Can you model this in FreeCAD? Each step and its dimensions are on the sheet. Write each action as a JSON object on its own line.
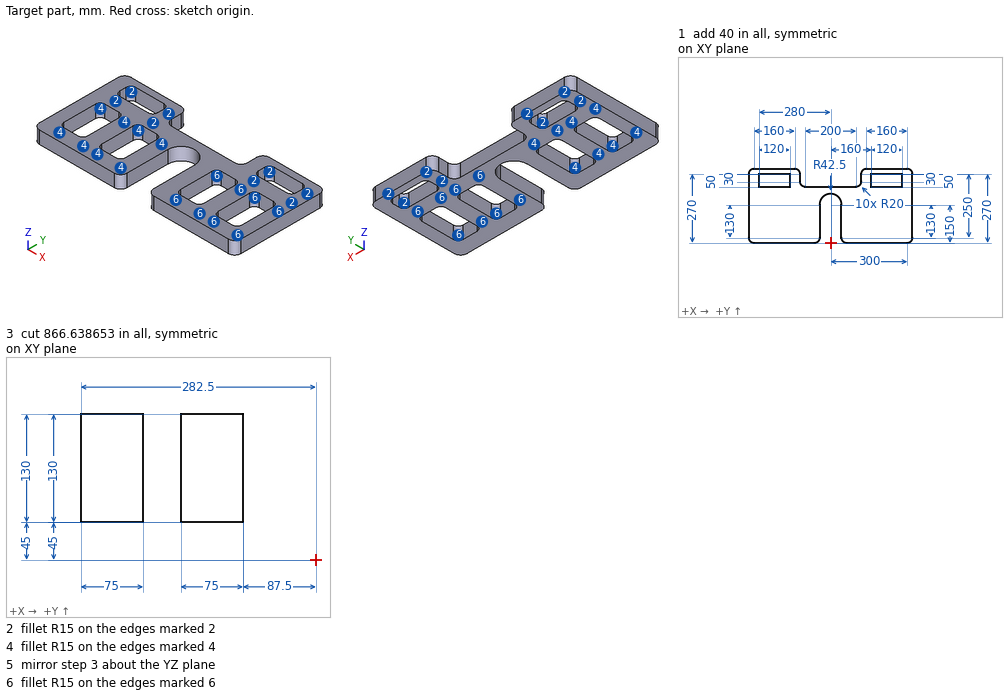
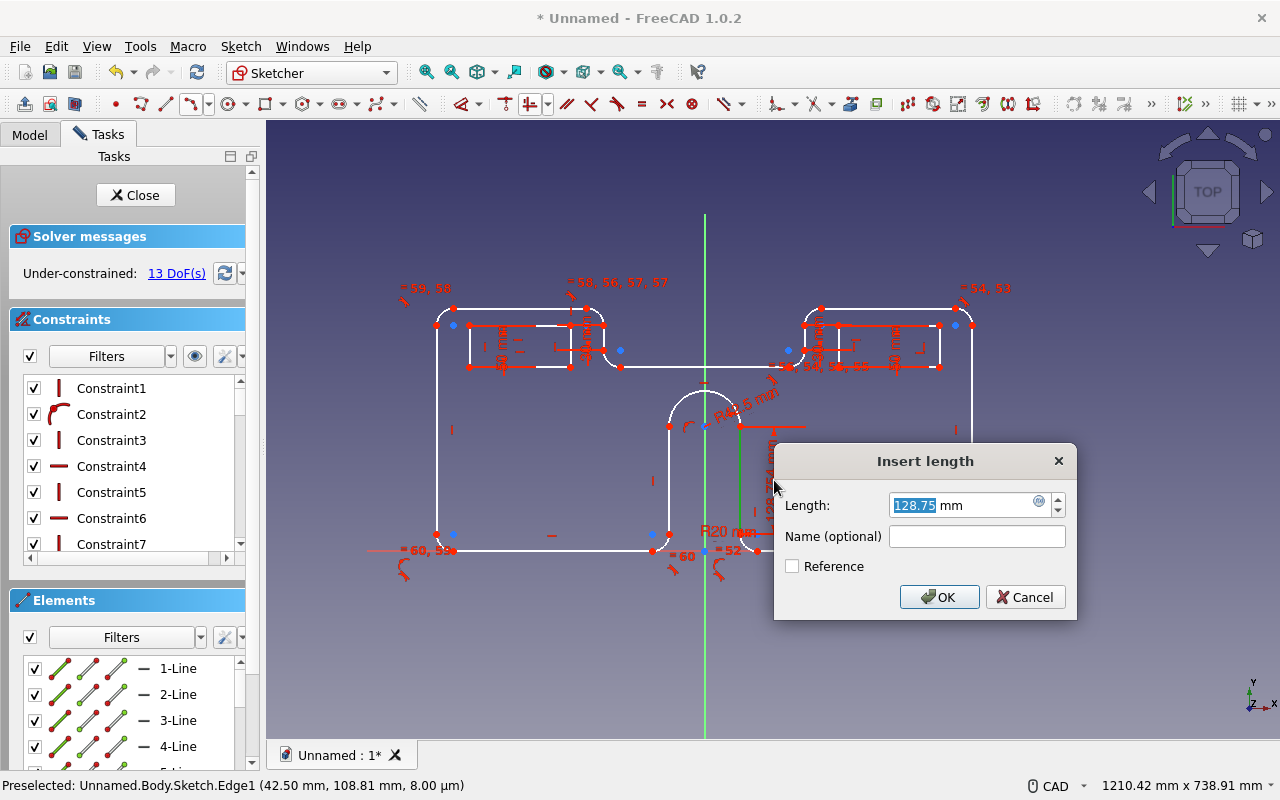
{"action": "type", "text": "130"}
{"action": "key", "text": "Return"}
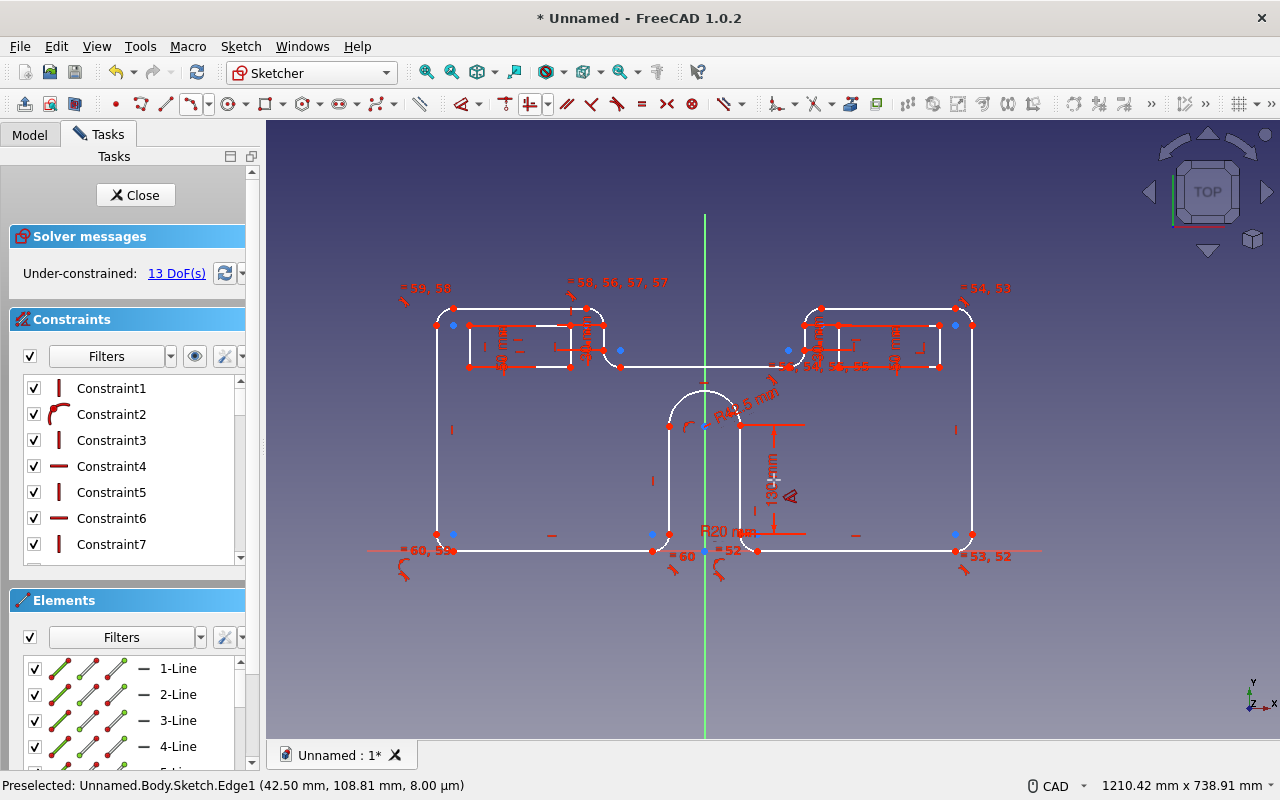
{"action": "left_click", "coordinate": [972, 472]}
{"action": "left_click", "coordinate": [1006, 430]}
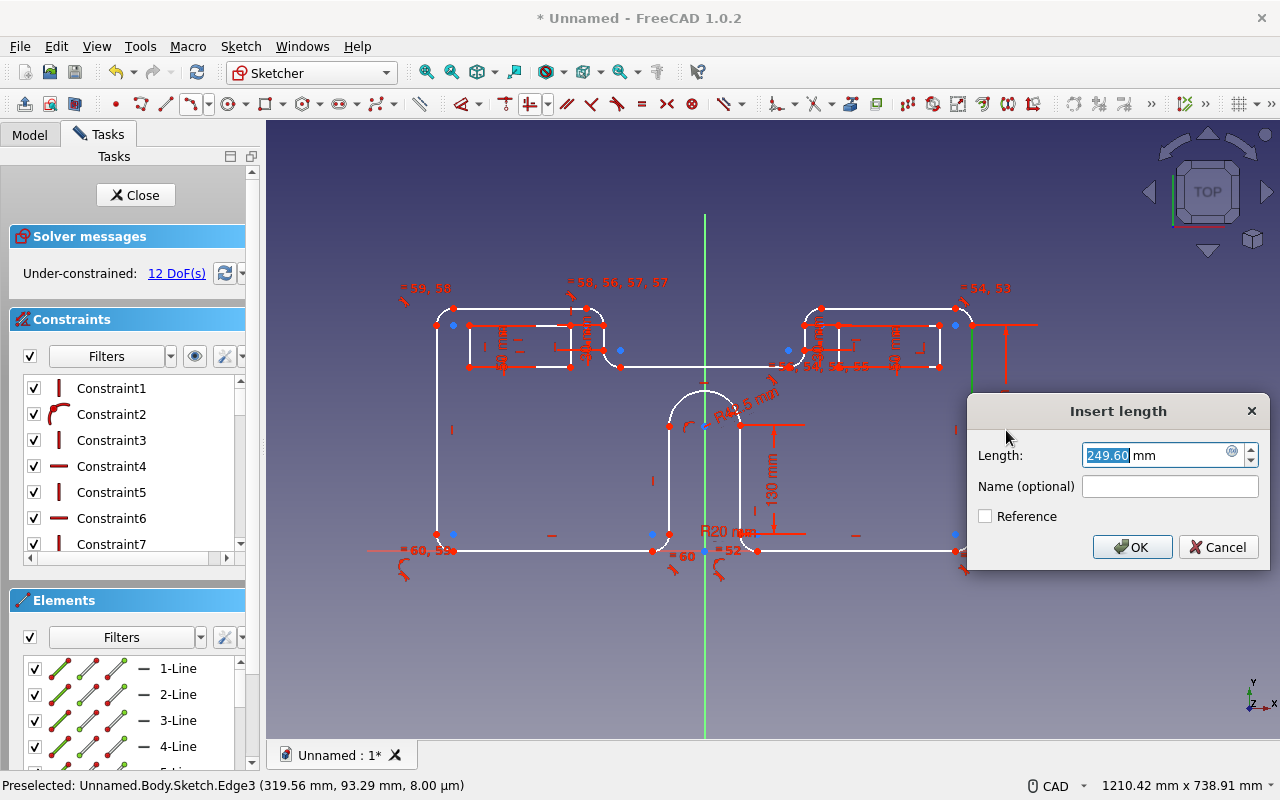
{"action": "type", "text": "250"}
{"action": "key", "text": "Return"}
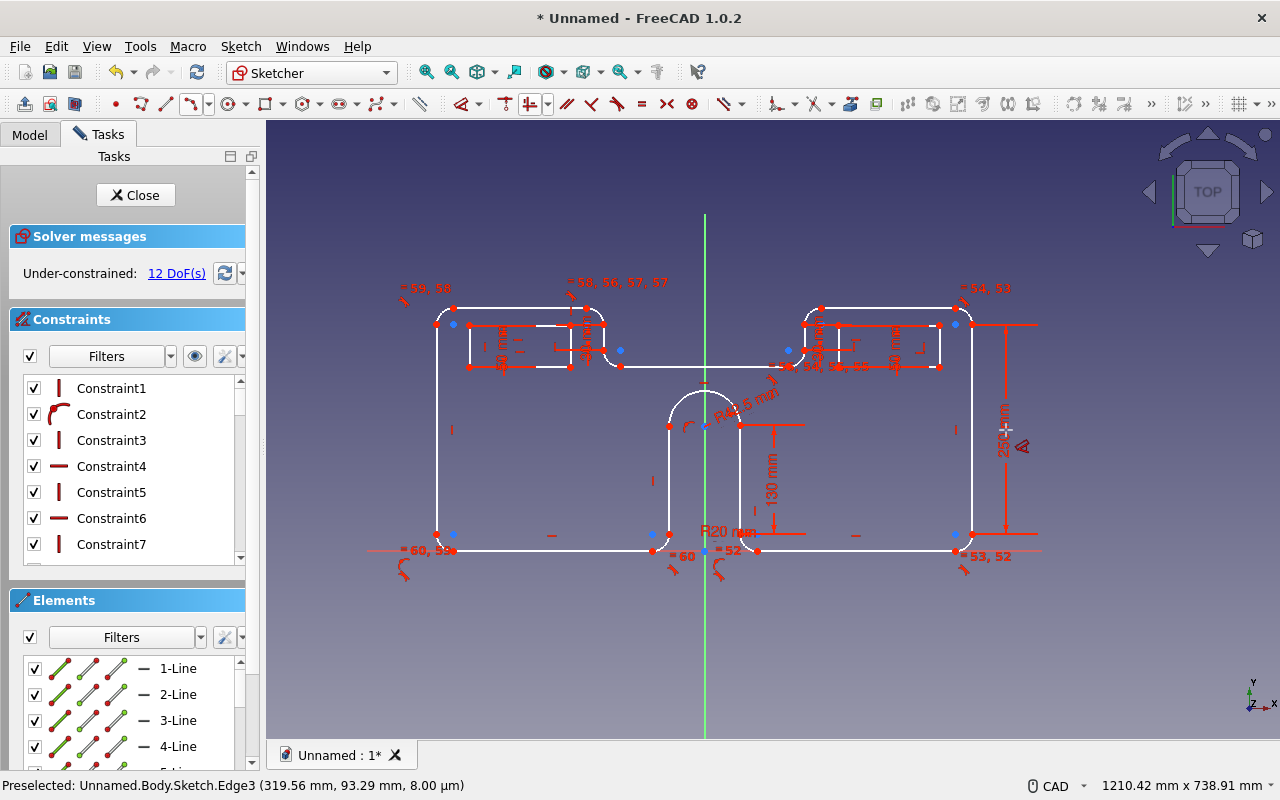
{"action": "left_click", "coordinate": [915, 308]}
{"action": "left_click", "coordinate": [889, 274]}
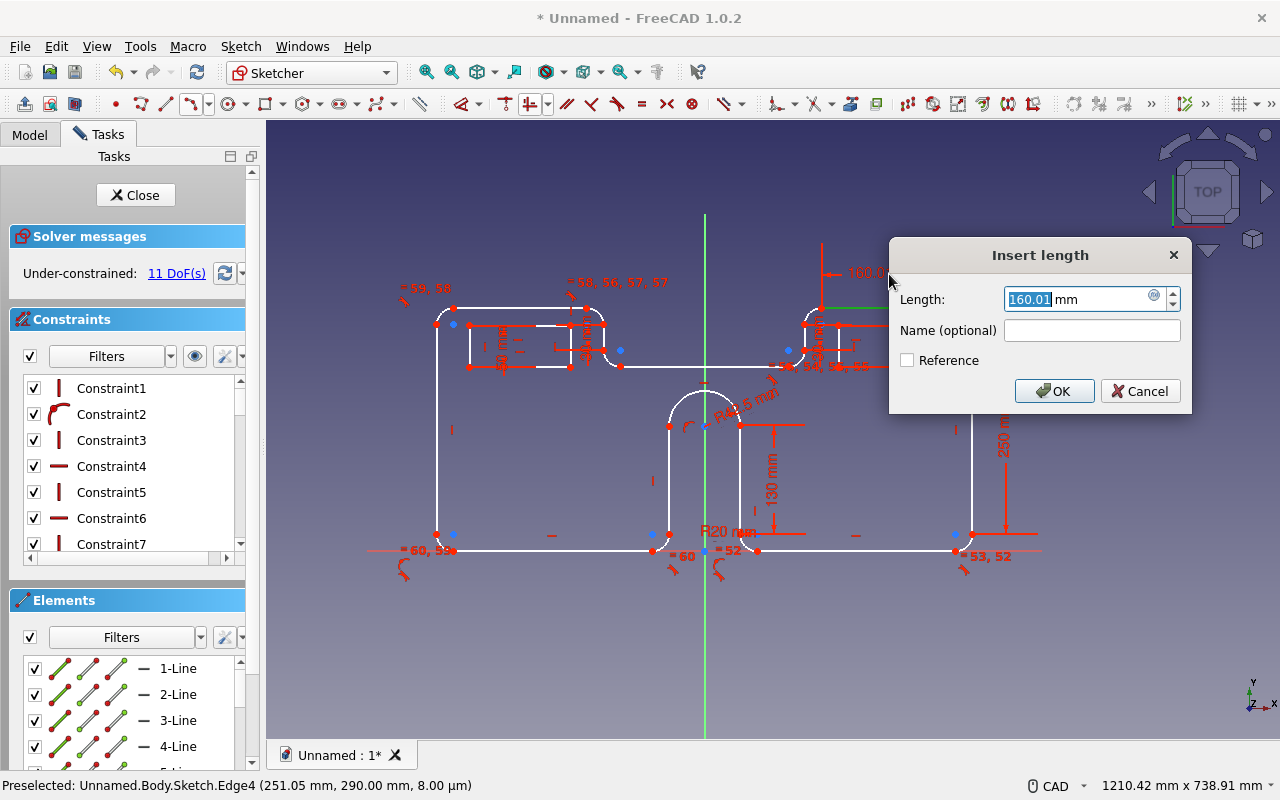
{"action": "type", "text": "160"}
{"action": "key", "text": "Return"}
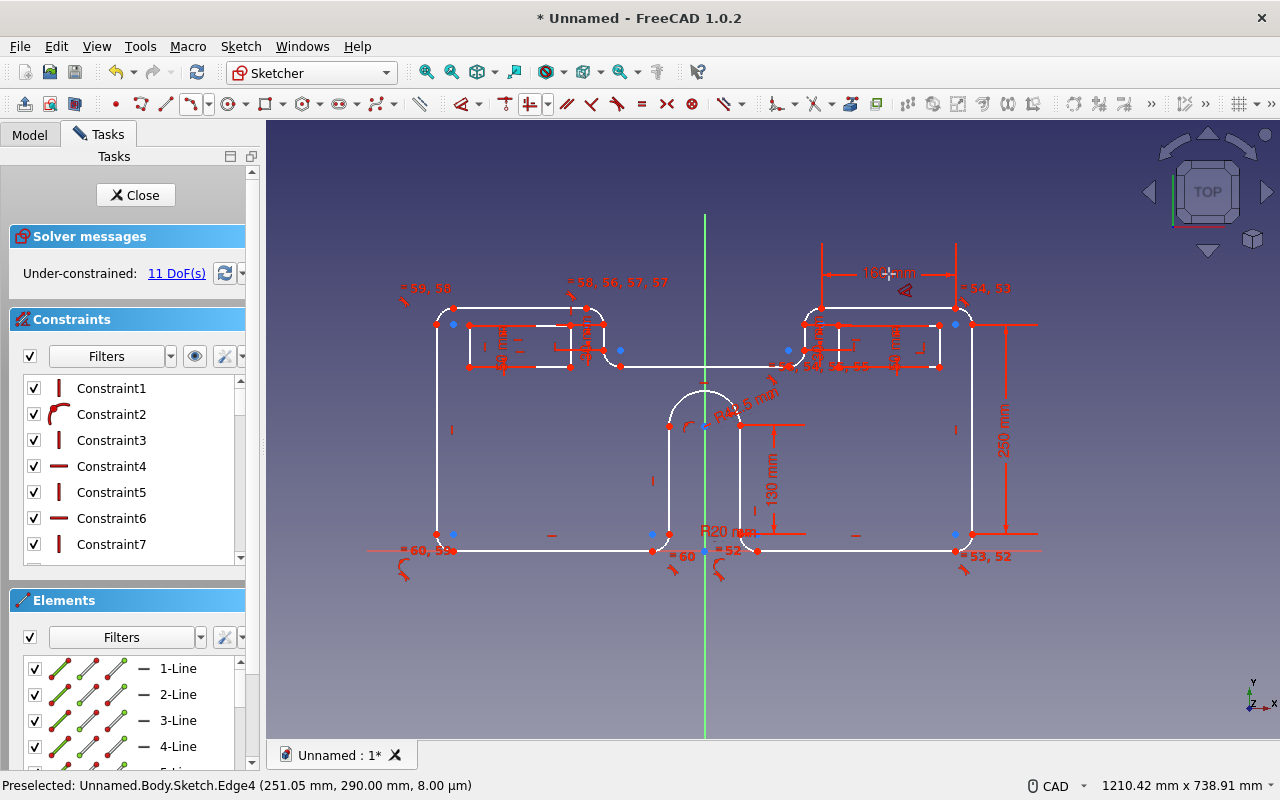
{"action": "left_click", "coordinate": [738, 367]}
{"action": "left_click", "coordinate": [666, 333]}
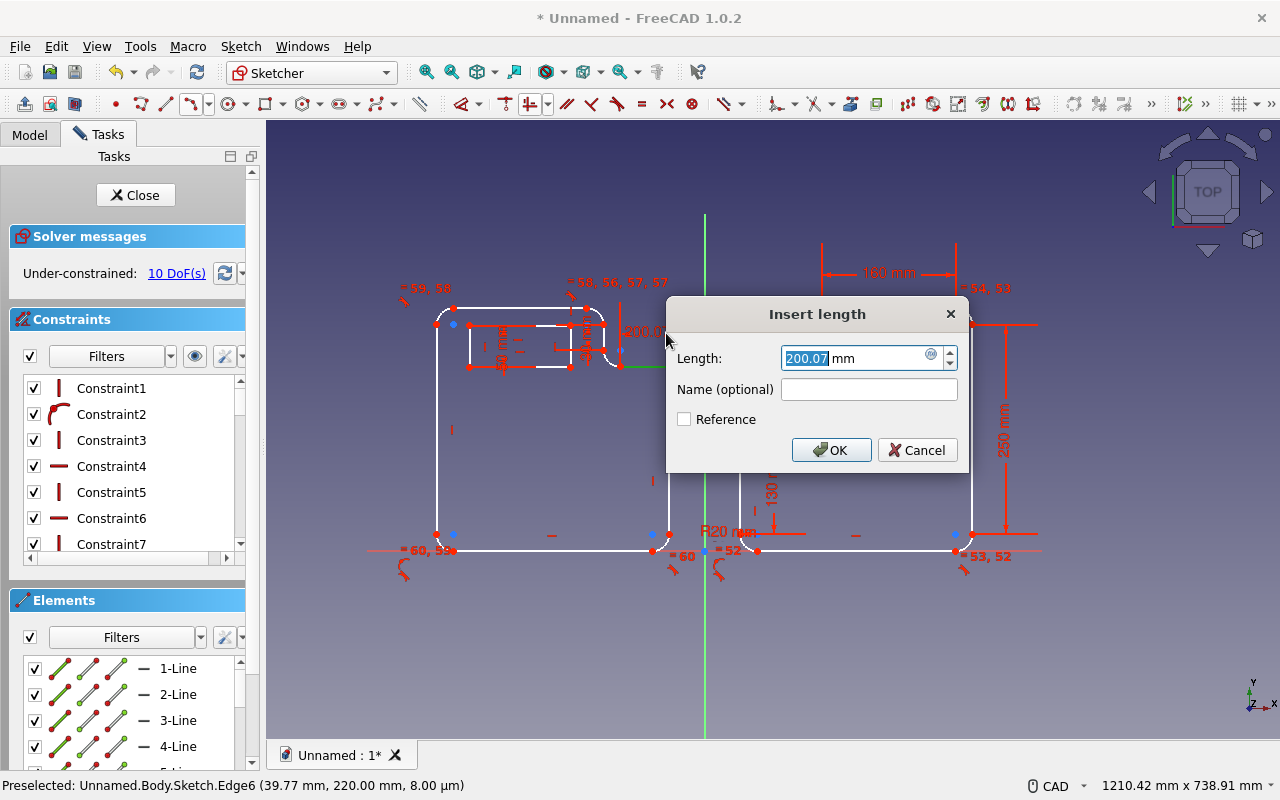
{"action": "type", "text": "200"}
{"action": "key", "text": "Return"}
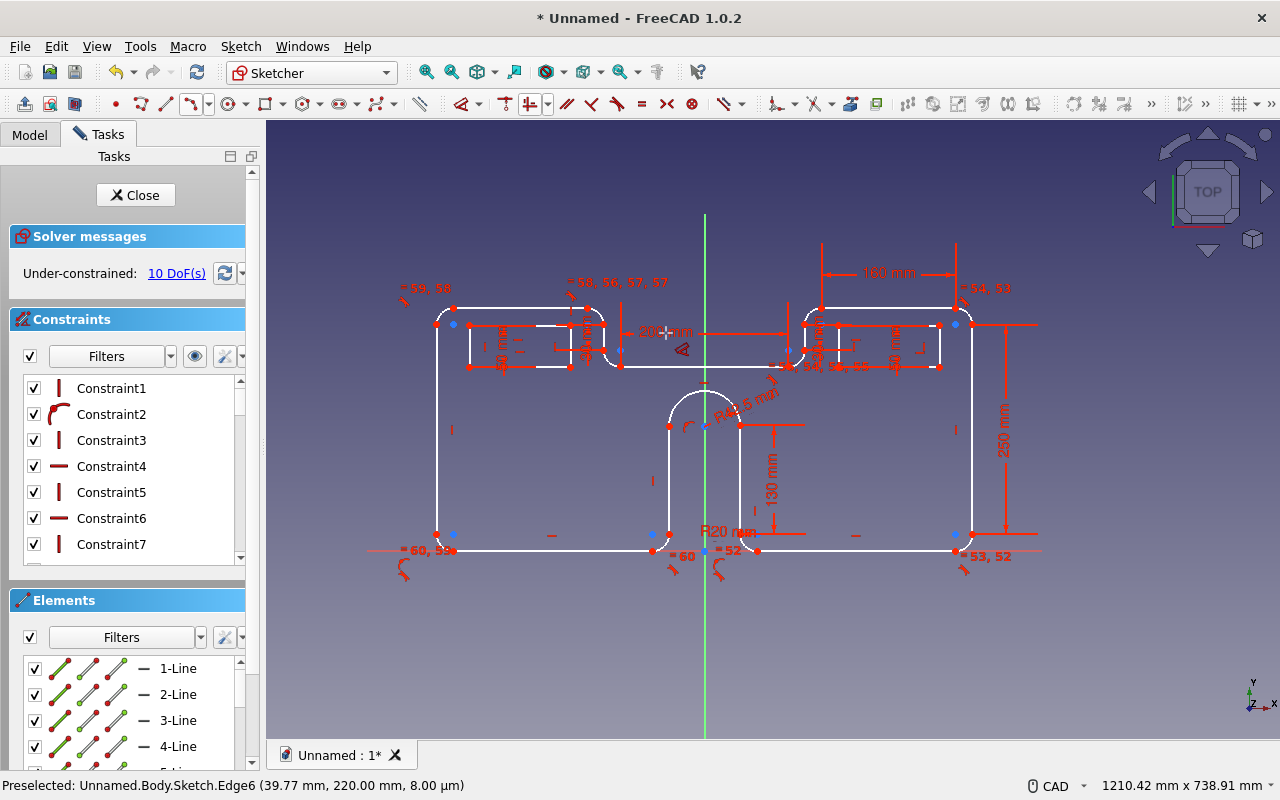
{"action": "left_click", "coordinate": [547, 308]}
{"action": "left_click", "coordinate": [520, 274]}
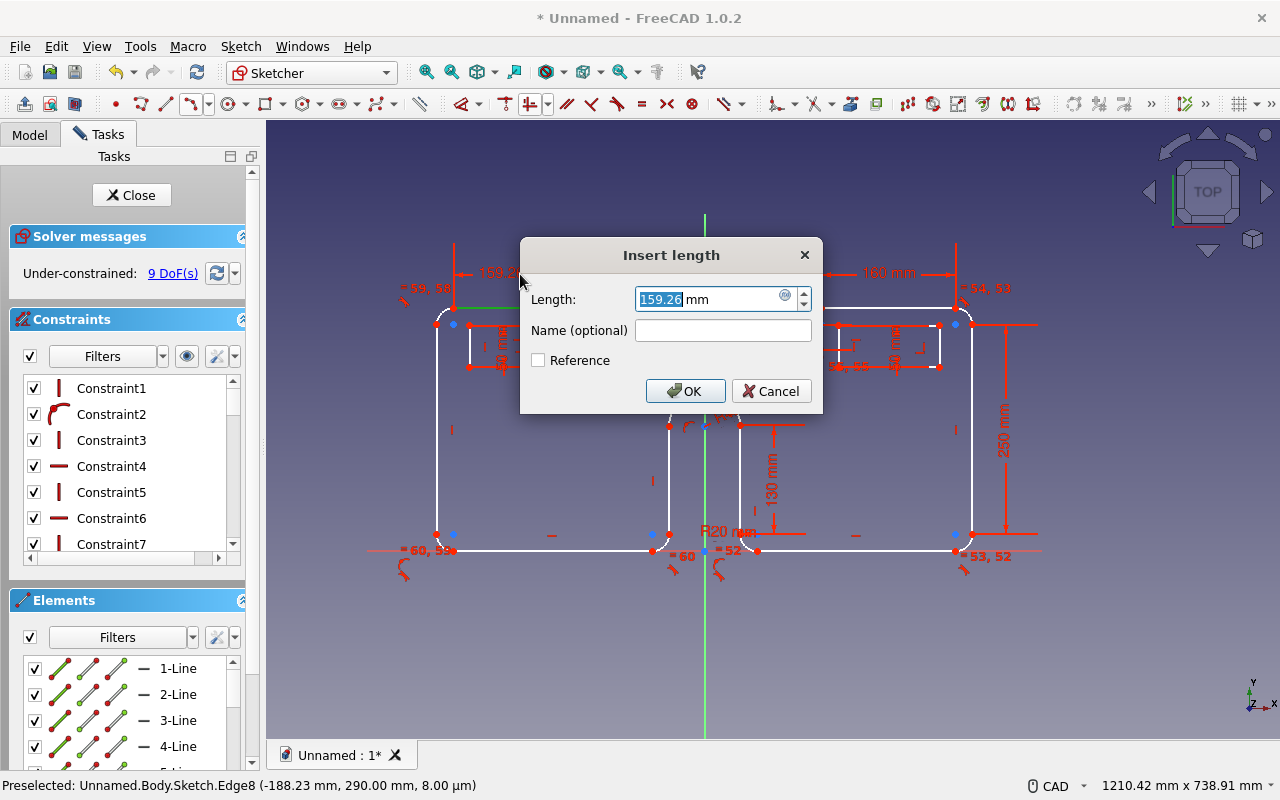
{"action": "type", "text": "160"}
{"action": "key", "text": "Return"}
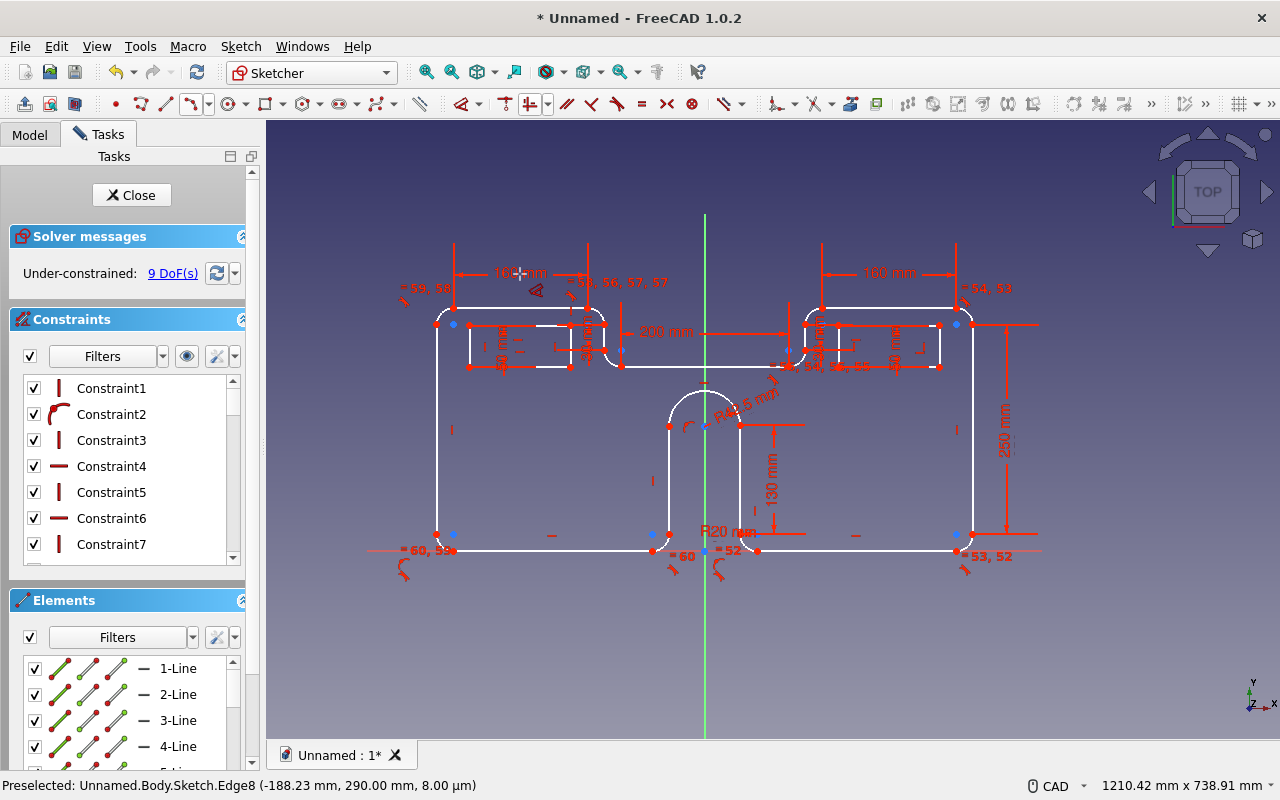
{"action": "left_click", "coordinate": [669, 502]}
{"action": "left_click", "coordinate": [635, 480]}